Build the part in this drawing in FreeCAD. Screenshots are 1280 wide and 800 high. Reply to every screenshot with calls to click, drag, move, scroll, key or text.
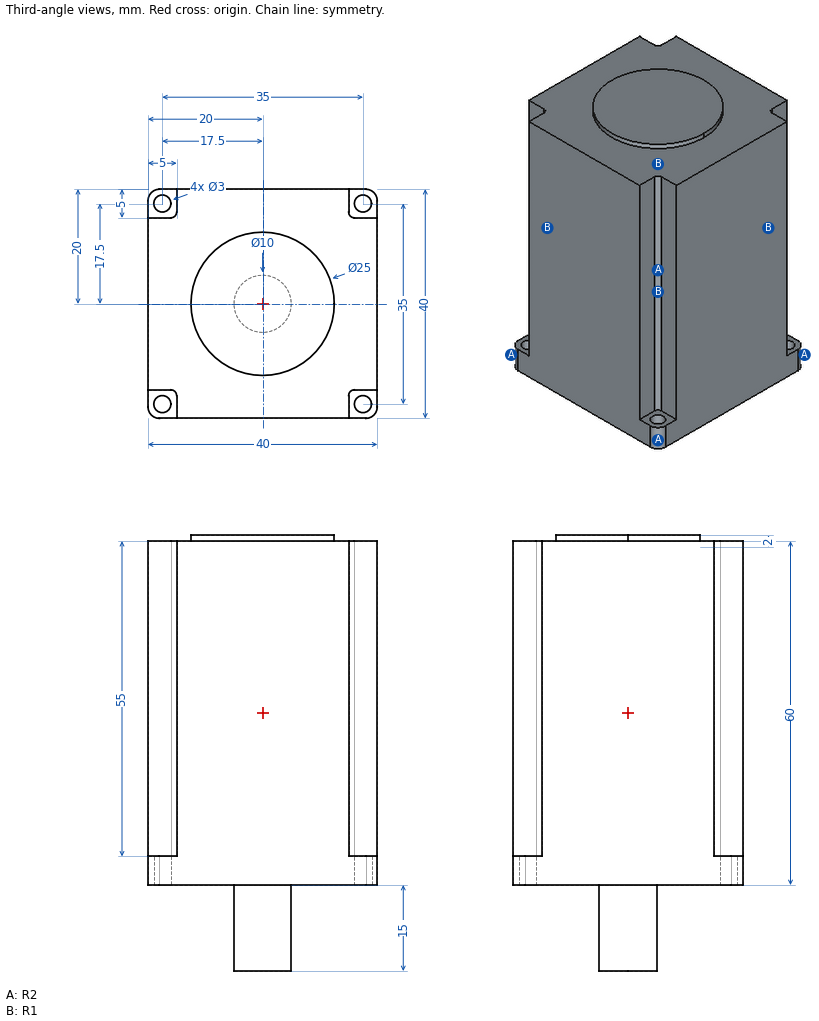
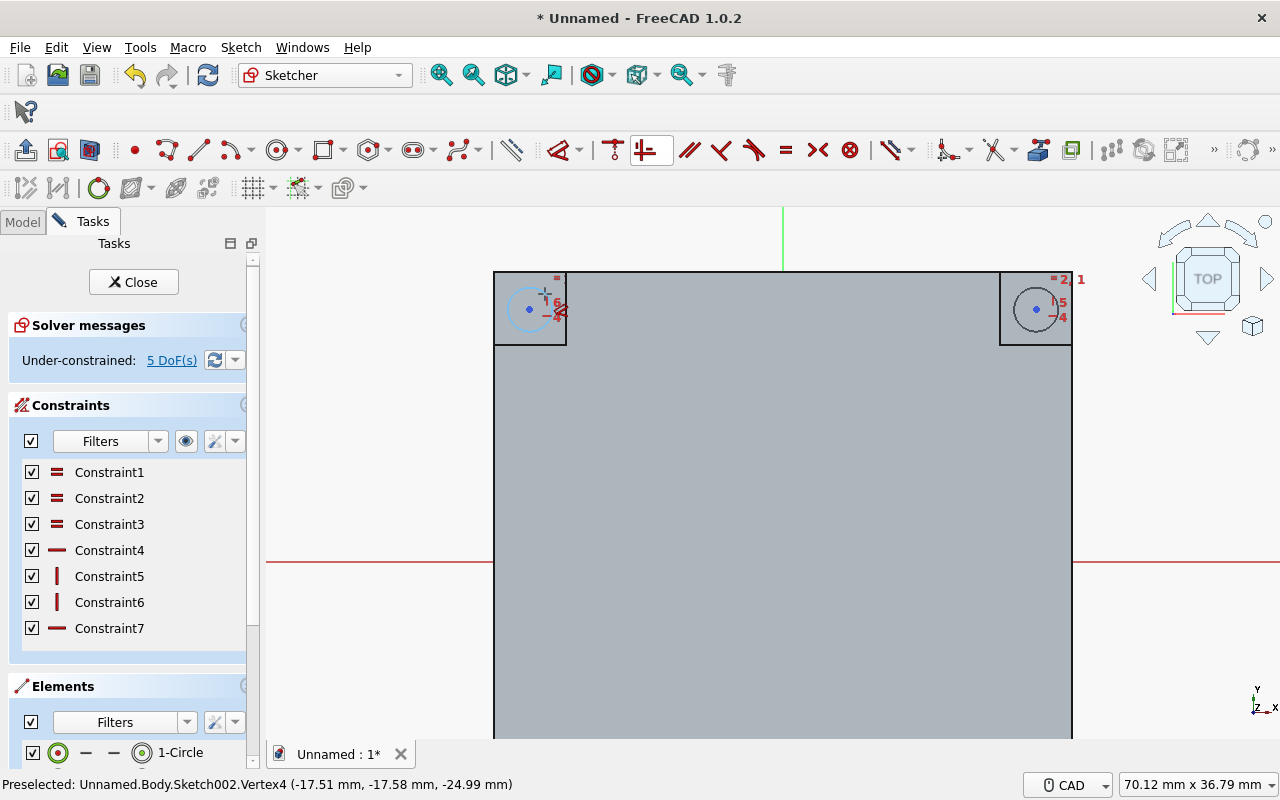
click(545, 294)
click(567, 271)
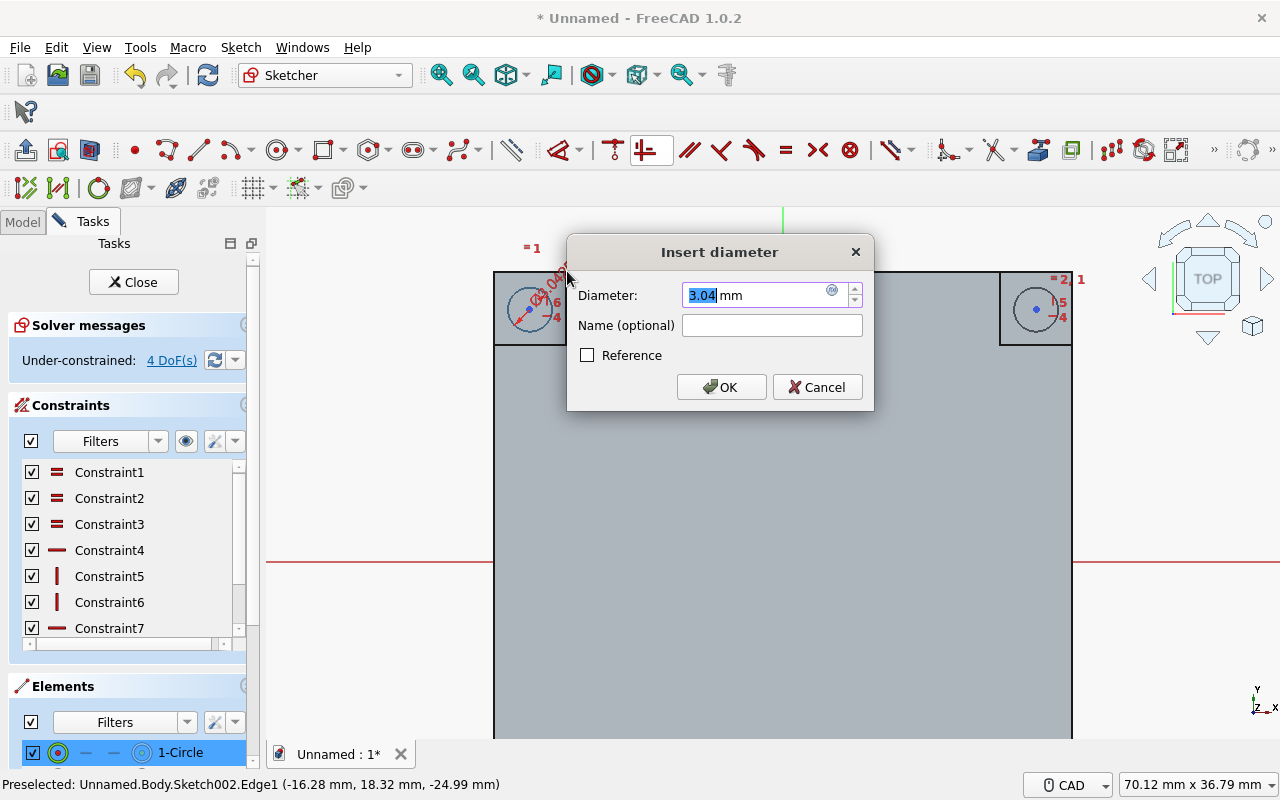
text(3)
key(Return)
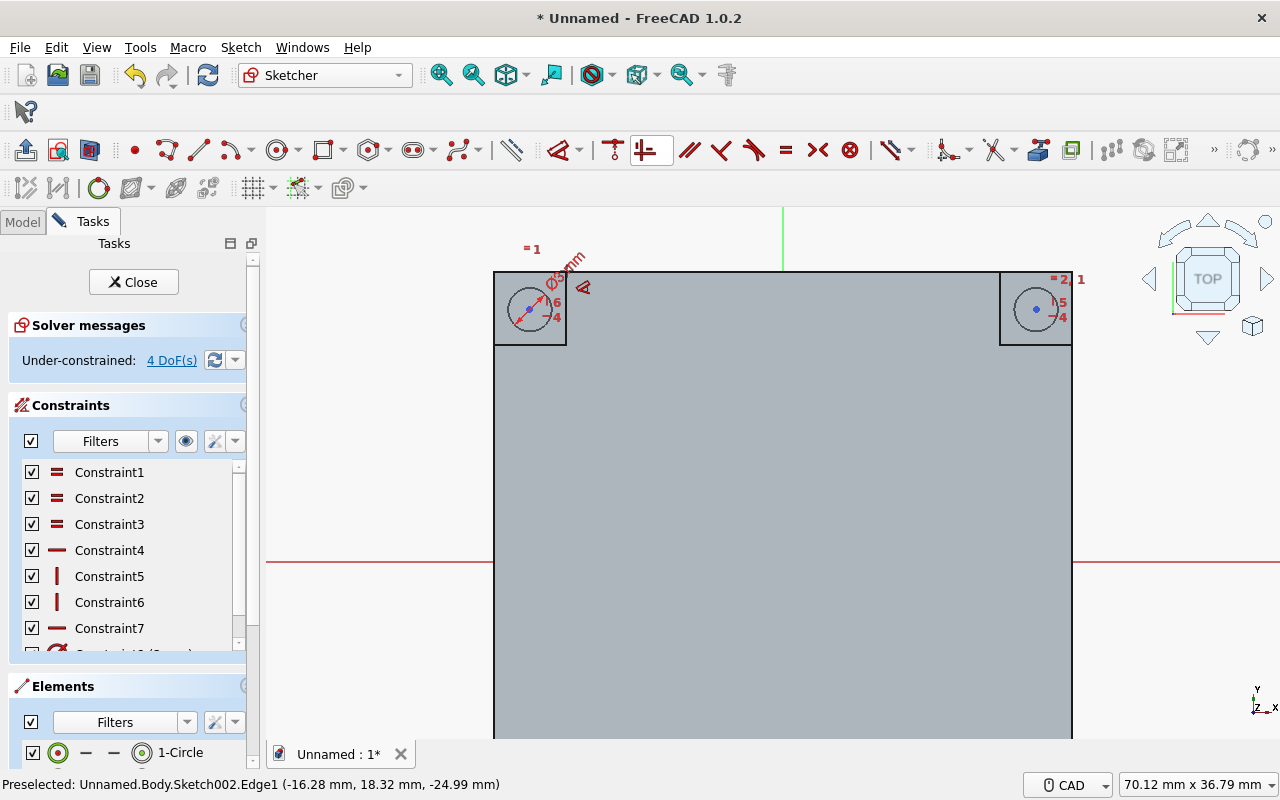
click(530, 310)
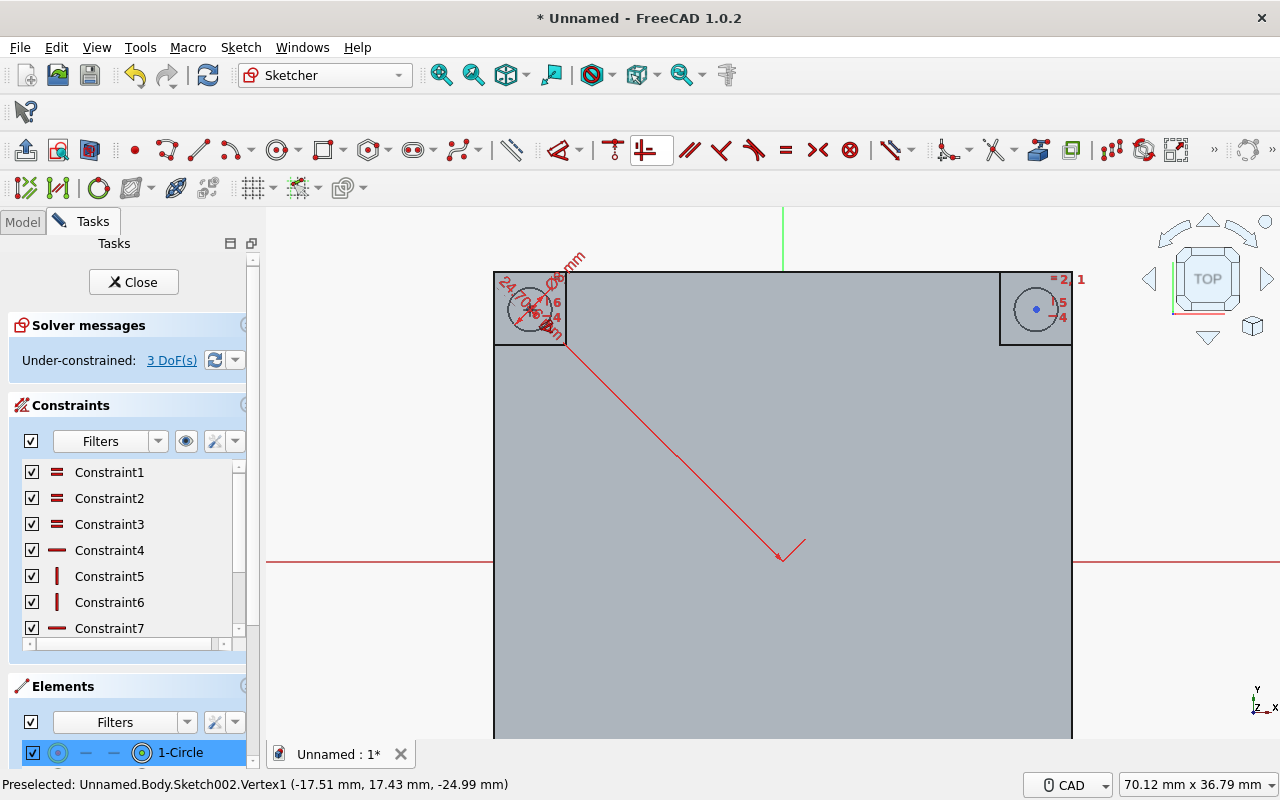
click(1036, 310)
click(667, 276)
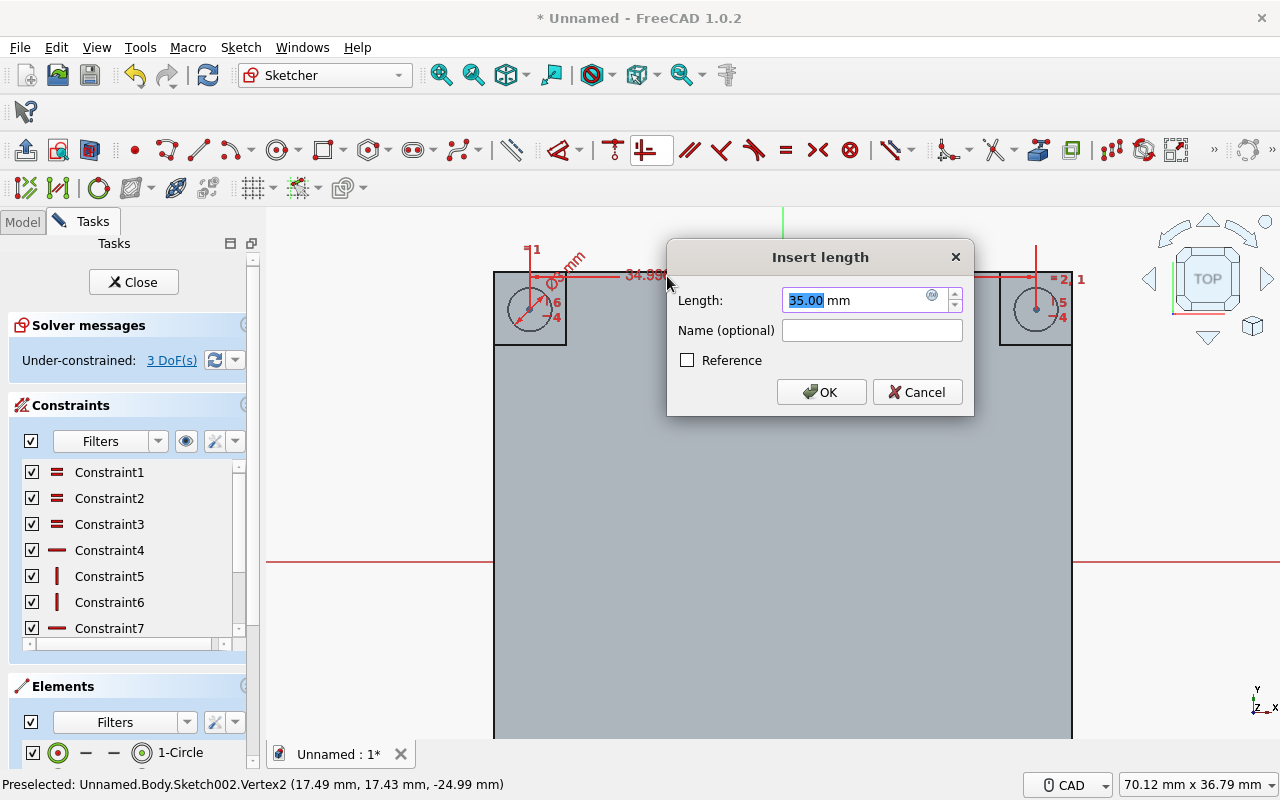
text(35)
key(Return)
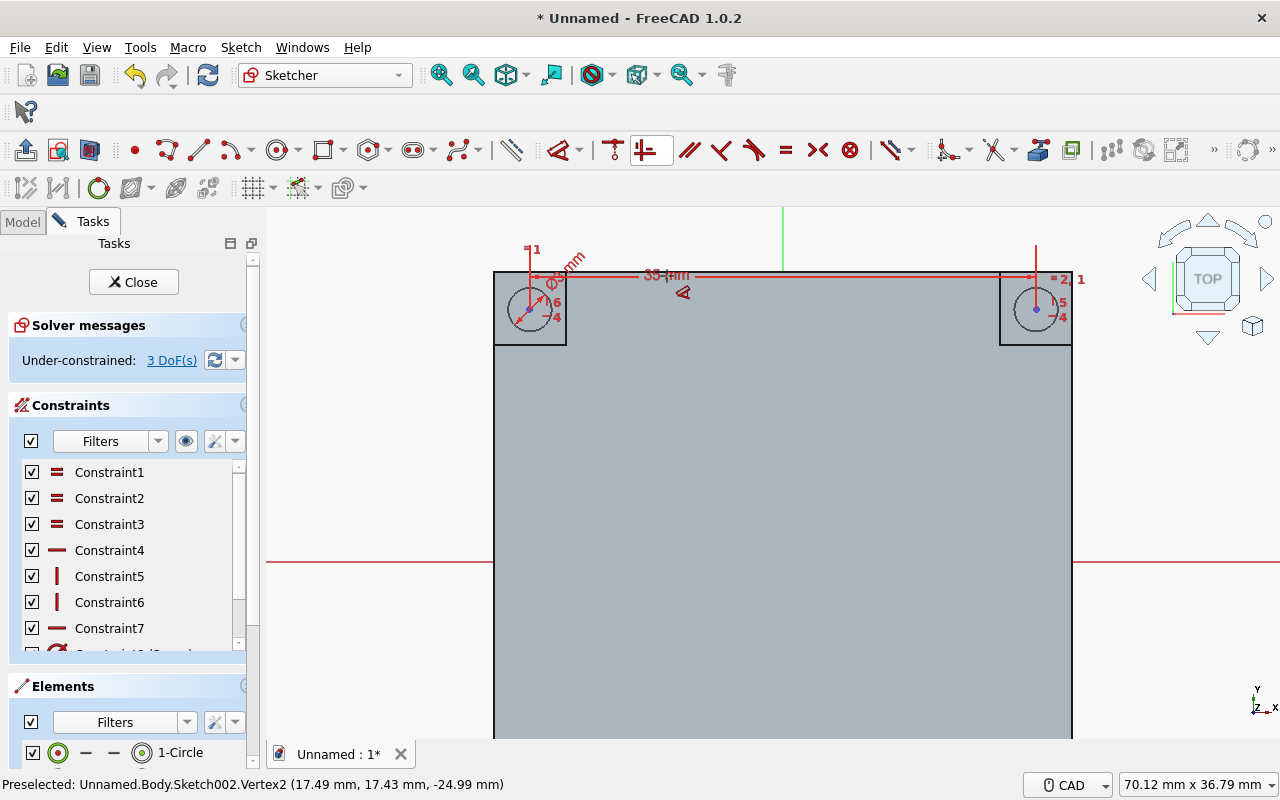
click(1036, 310)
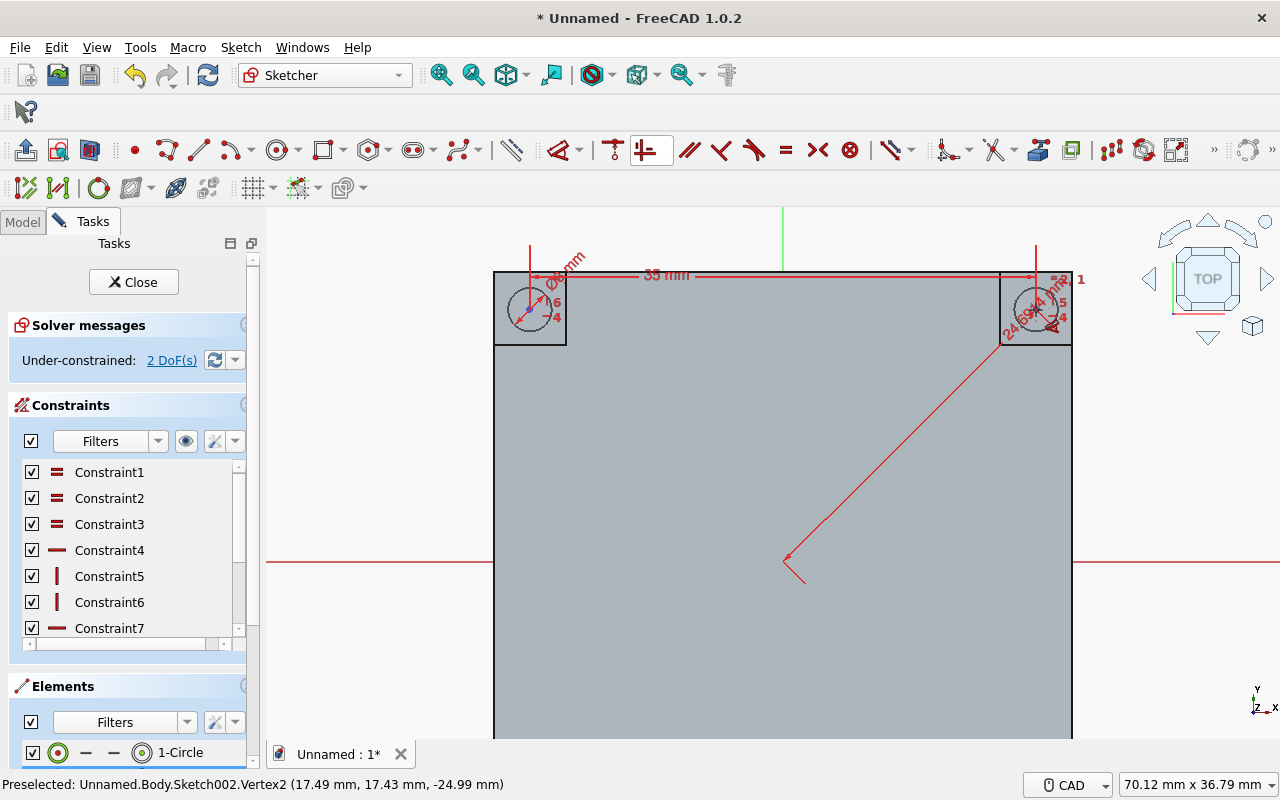
scroll(545, 293, down, 2)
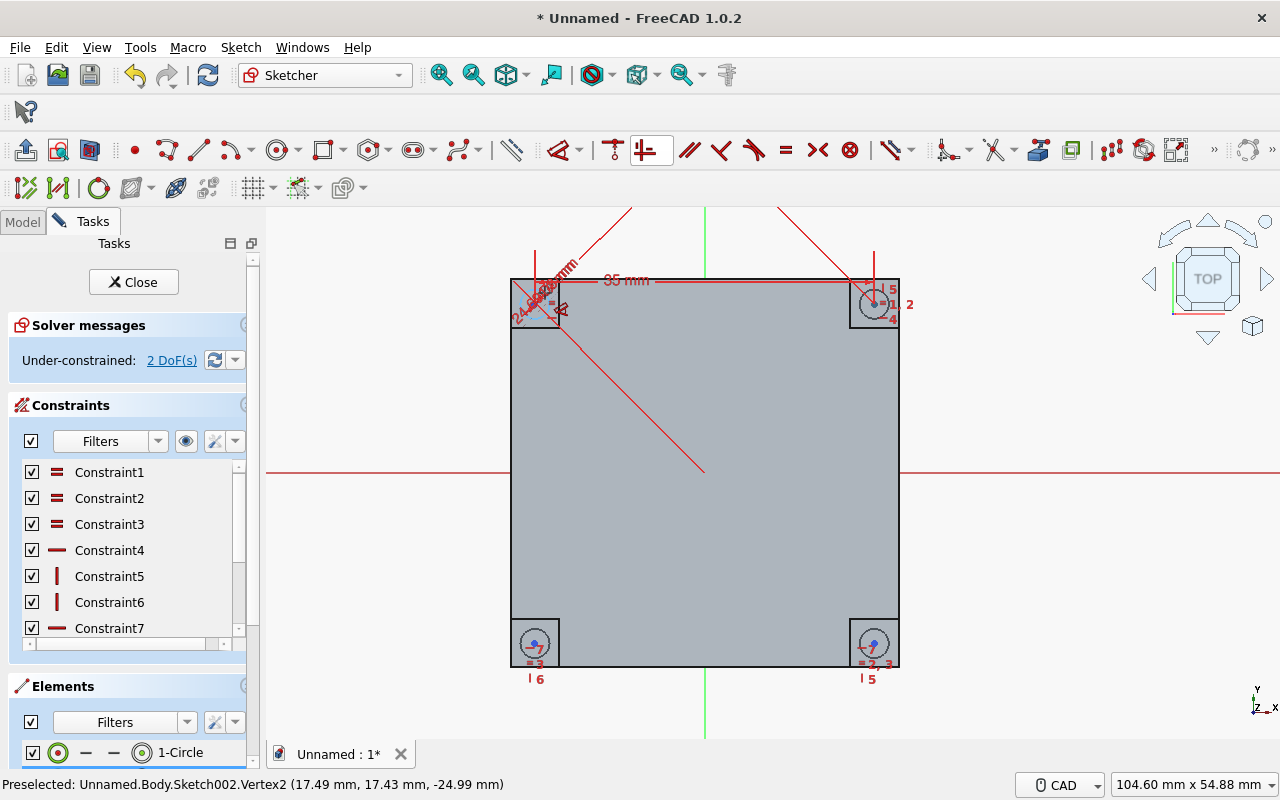
click(874, 643)
click(908, 396)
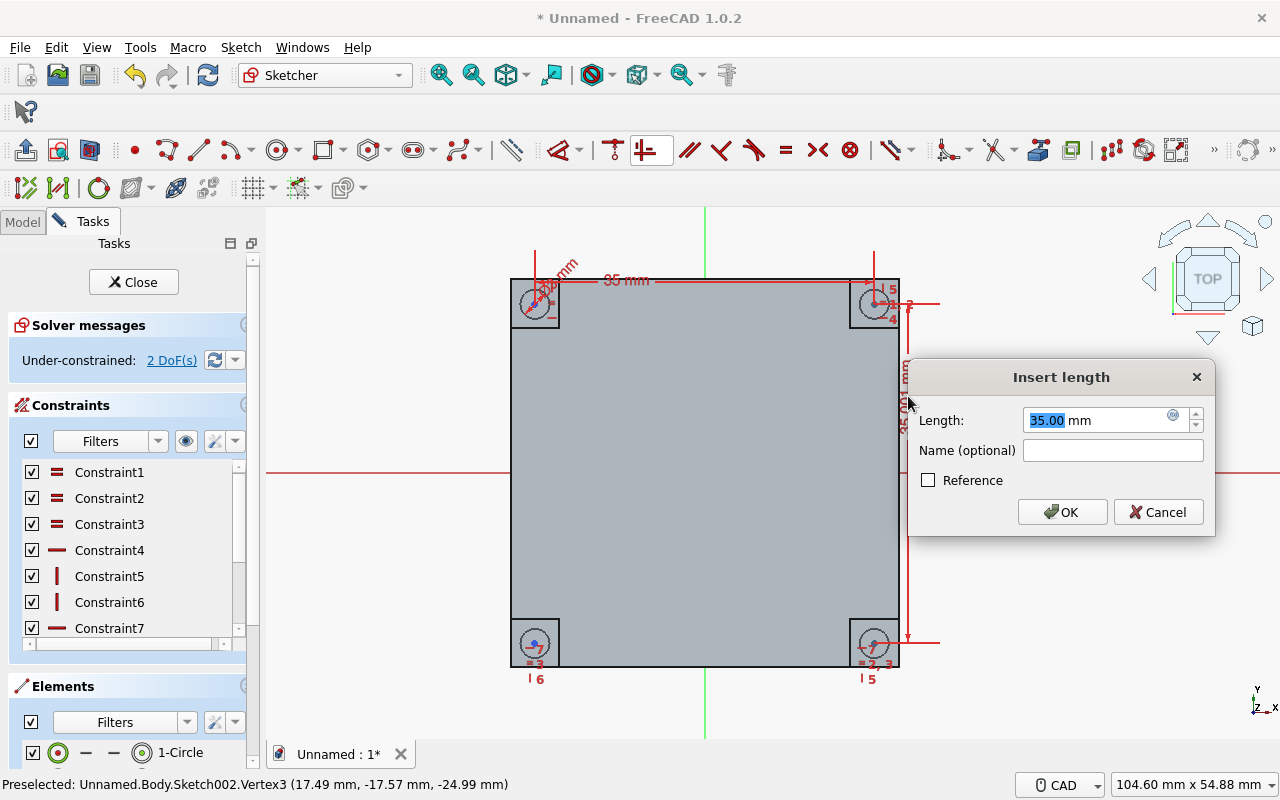
text(35)
key(Return)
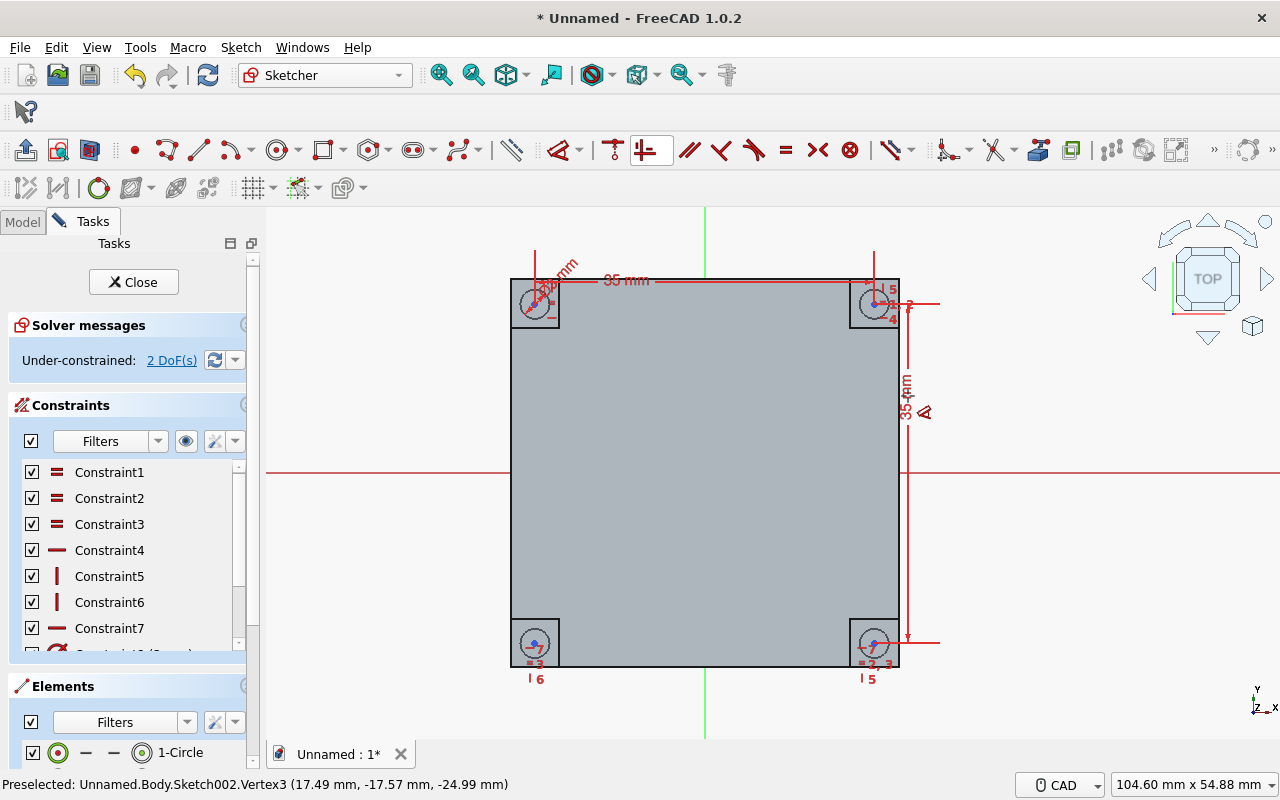
click(535, 304)
click(620, 507)